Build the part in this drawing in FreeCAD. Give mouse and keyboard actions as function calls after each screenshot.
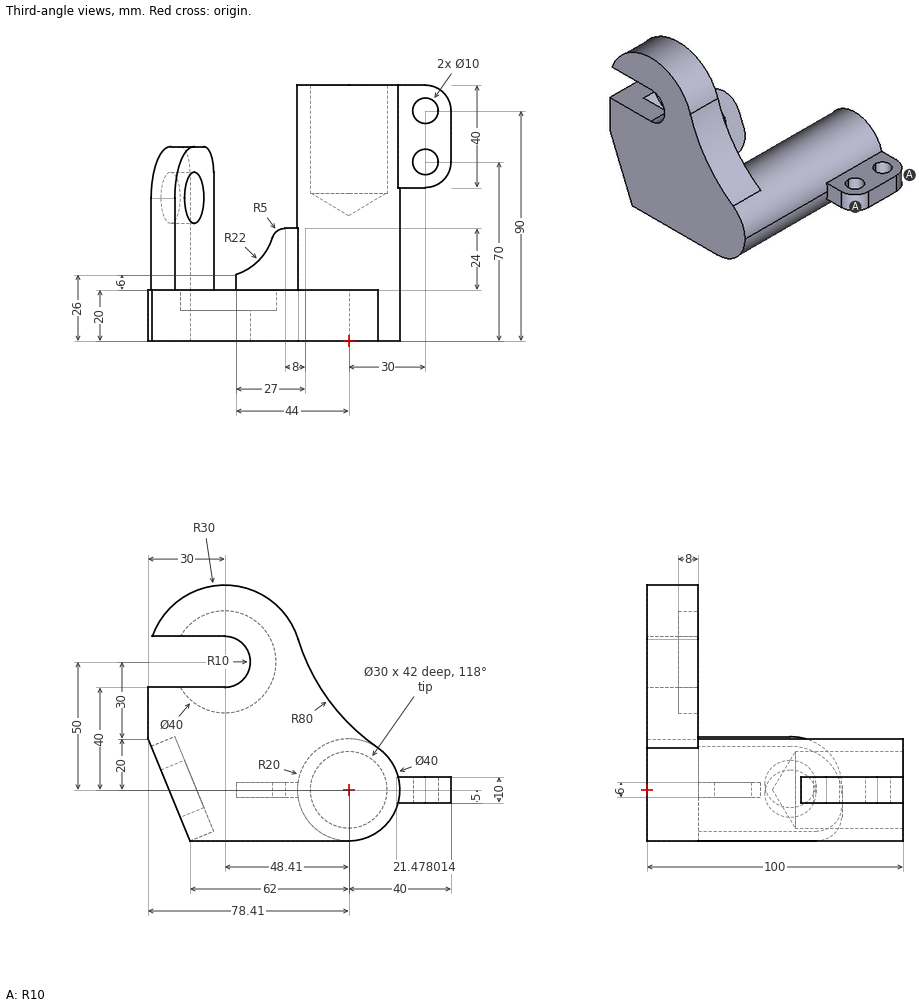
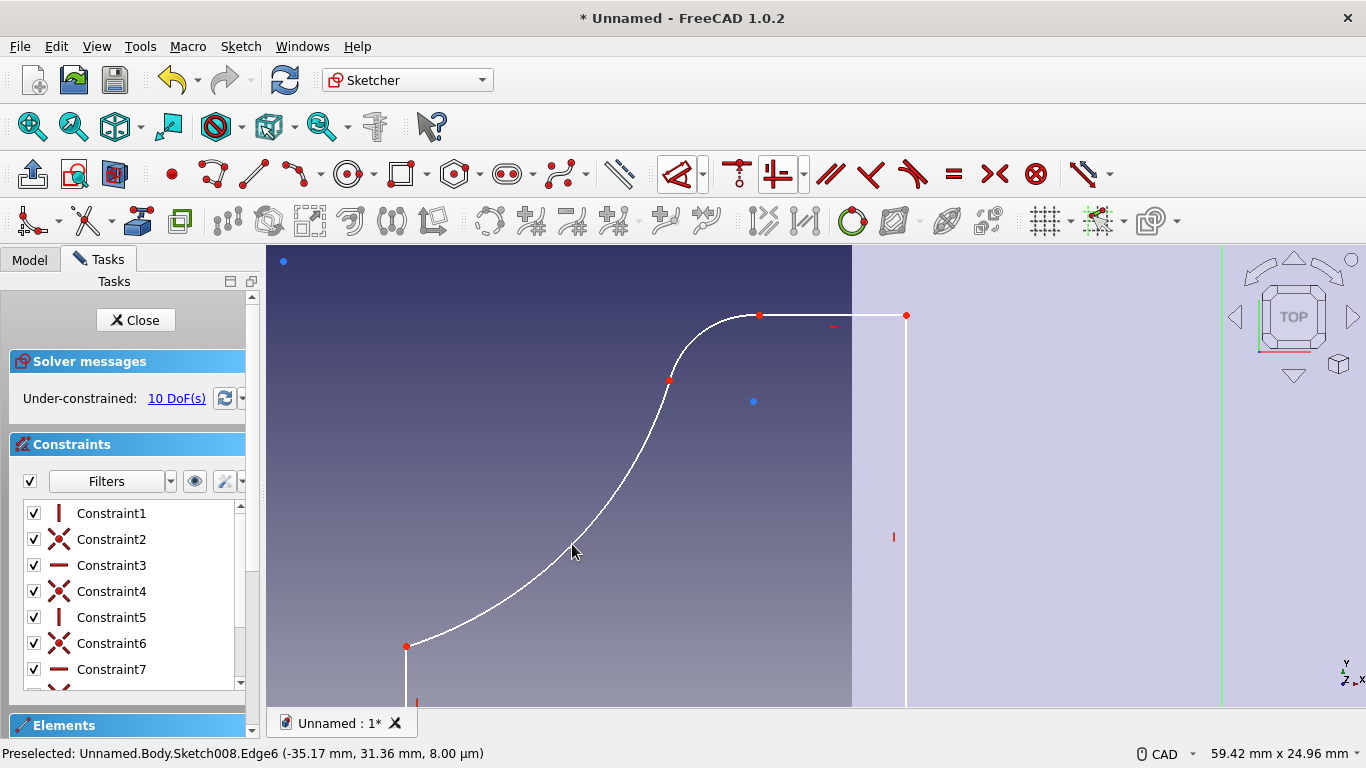
click(862, 315)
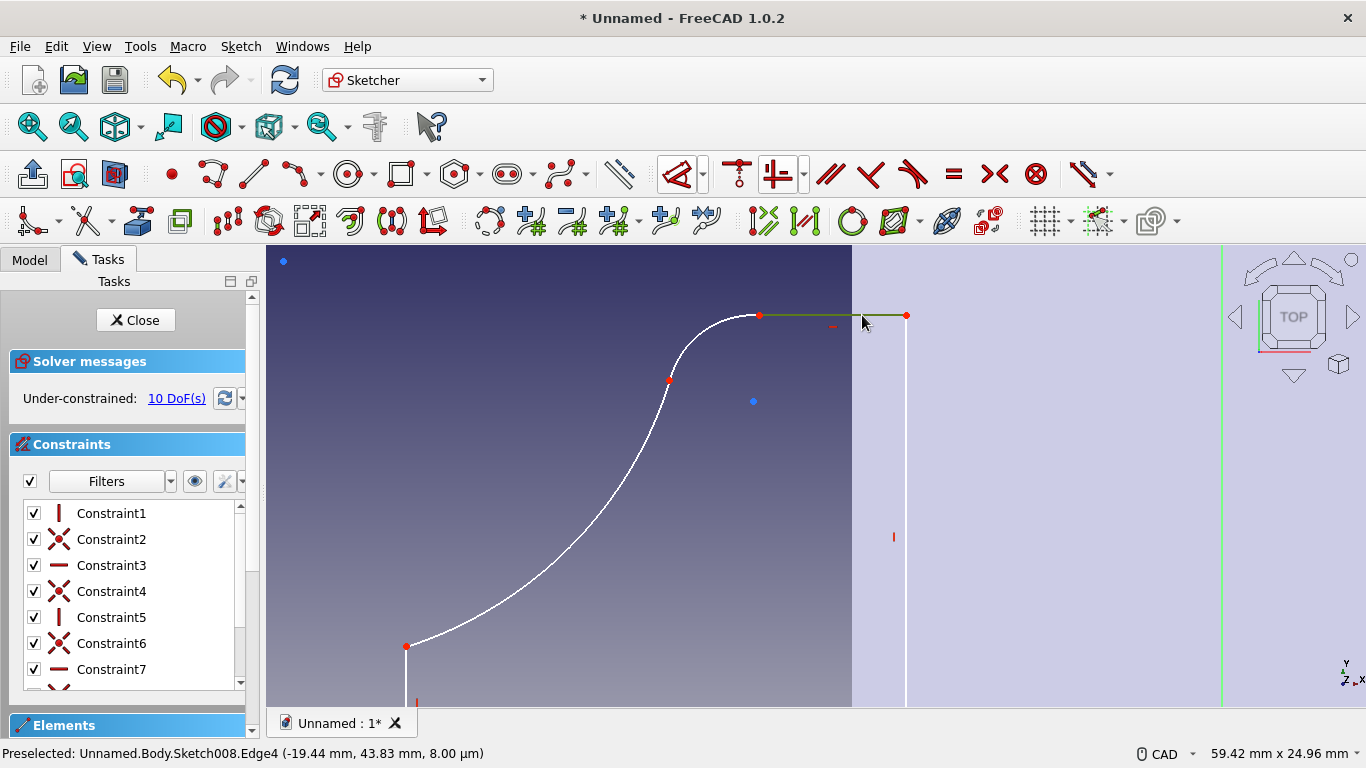
click(724, 320)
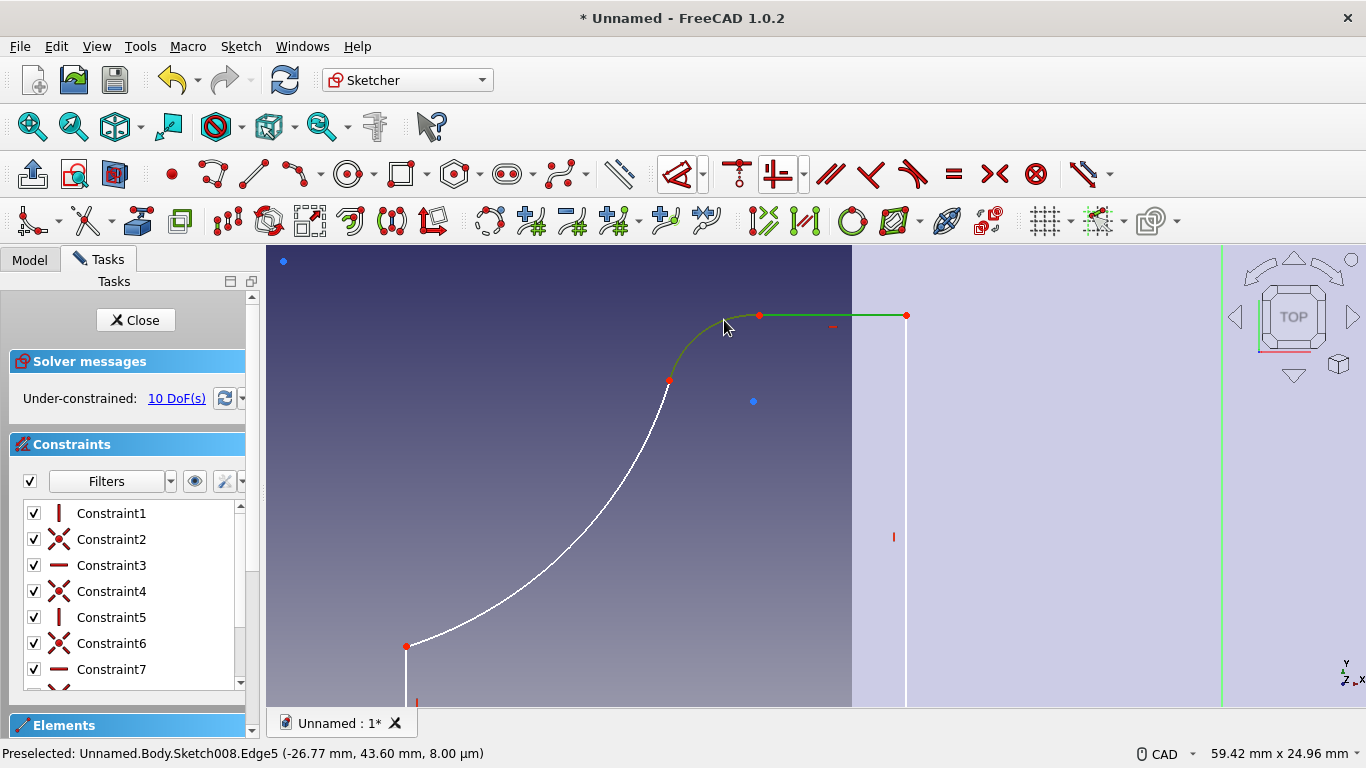
key(t)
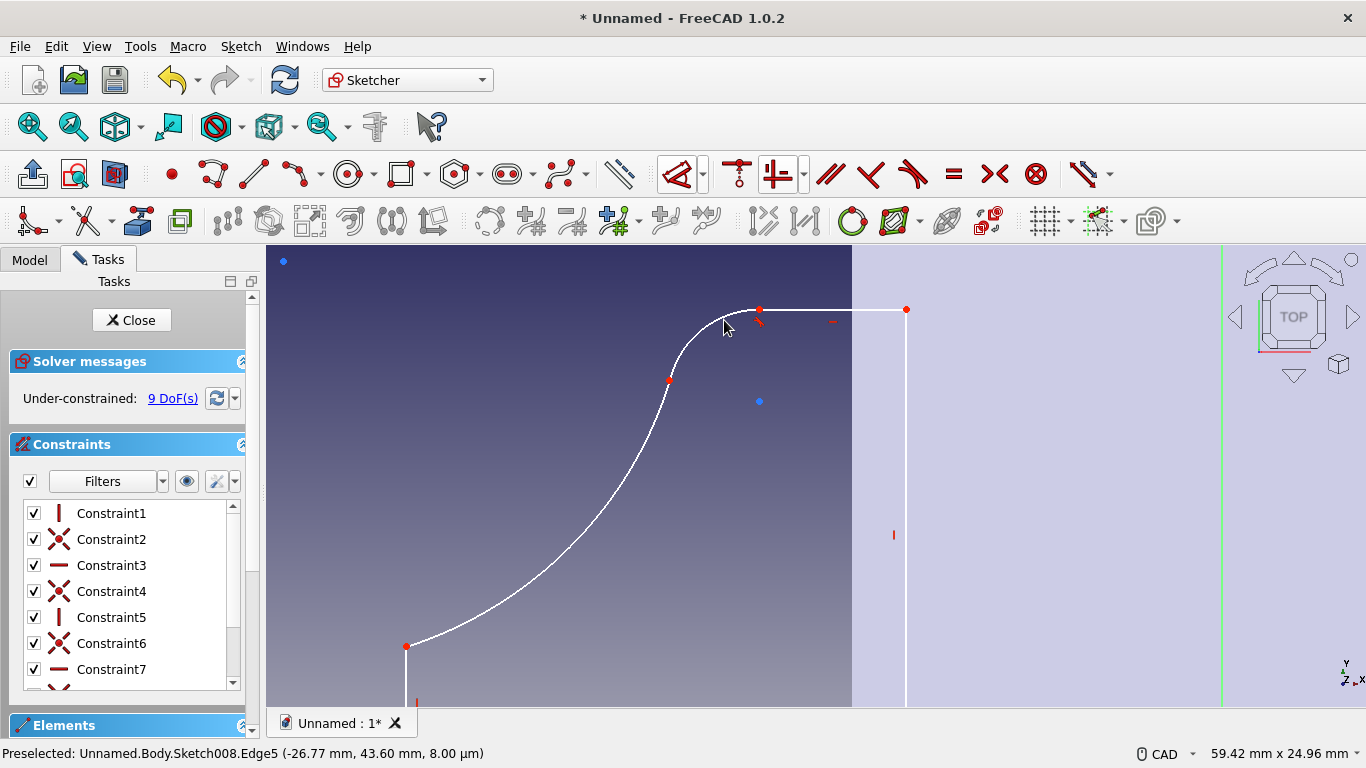
click(724, 317)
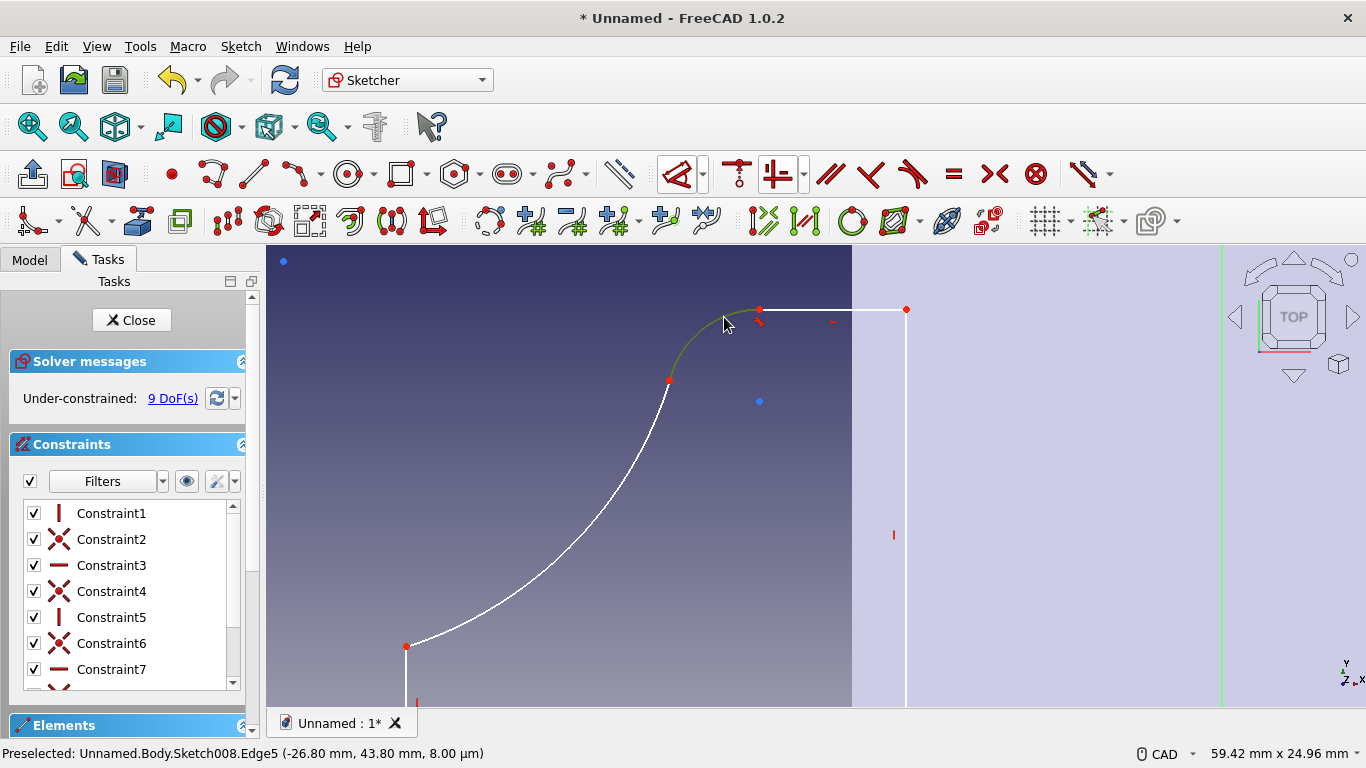
click(511, 596)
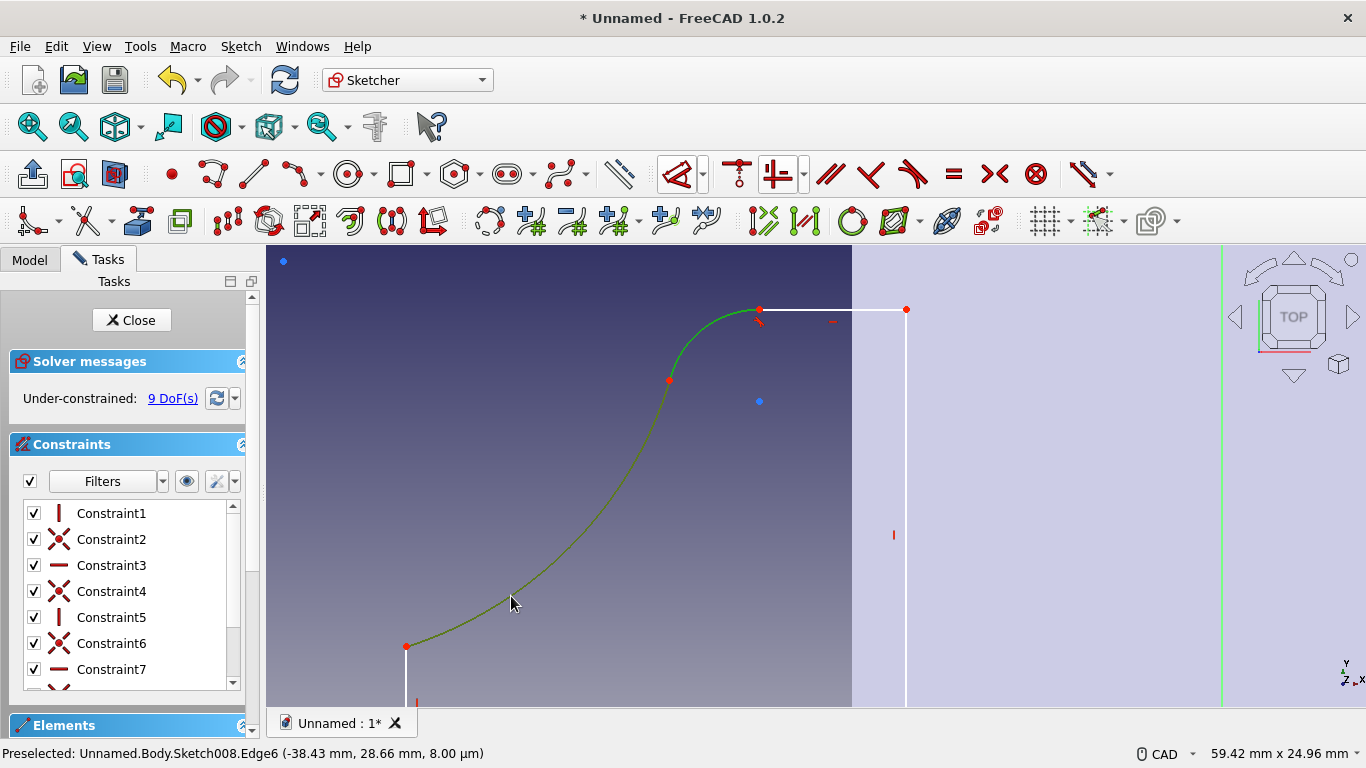
click(913, 174)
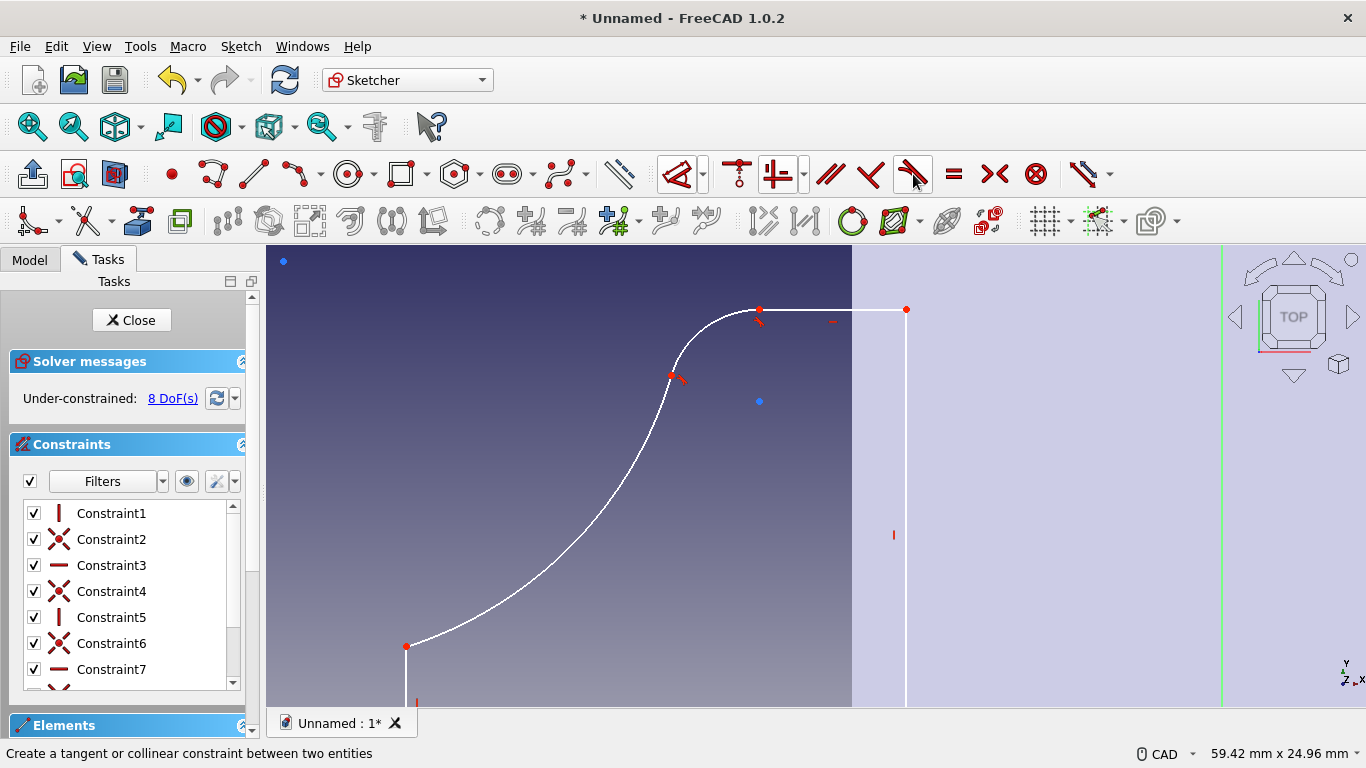
key(d)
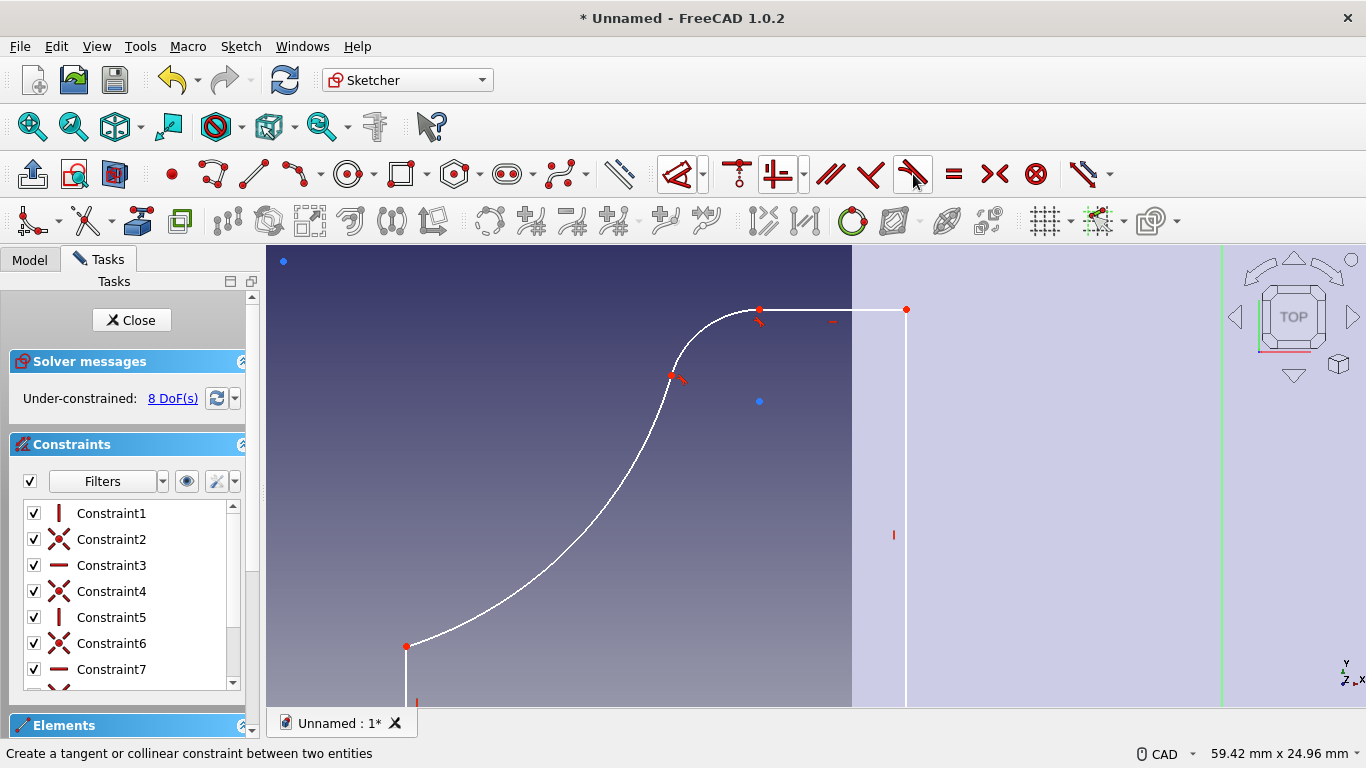
click(725, 317)
click(713, 287)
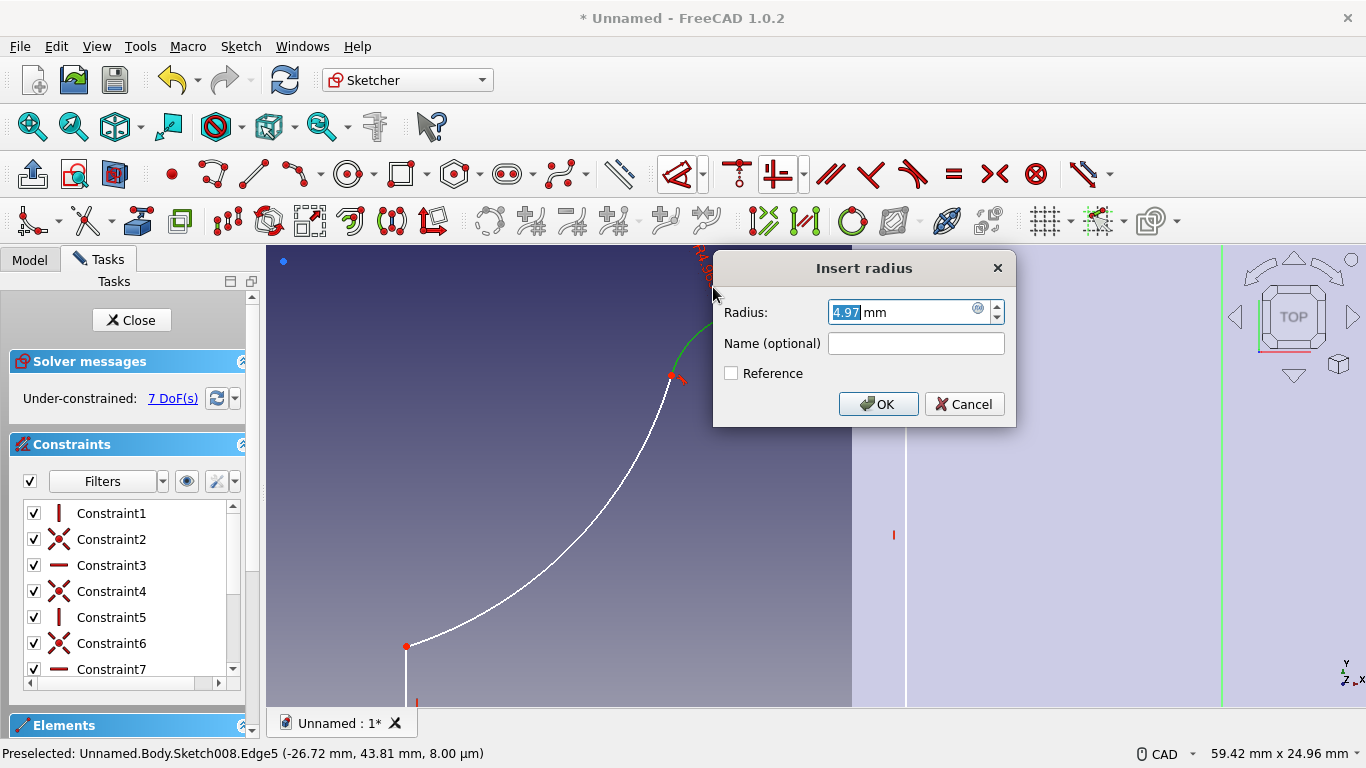
text(5)
key(Return)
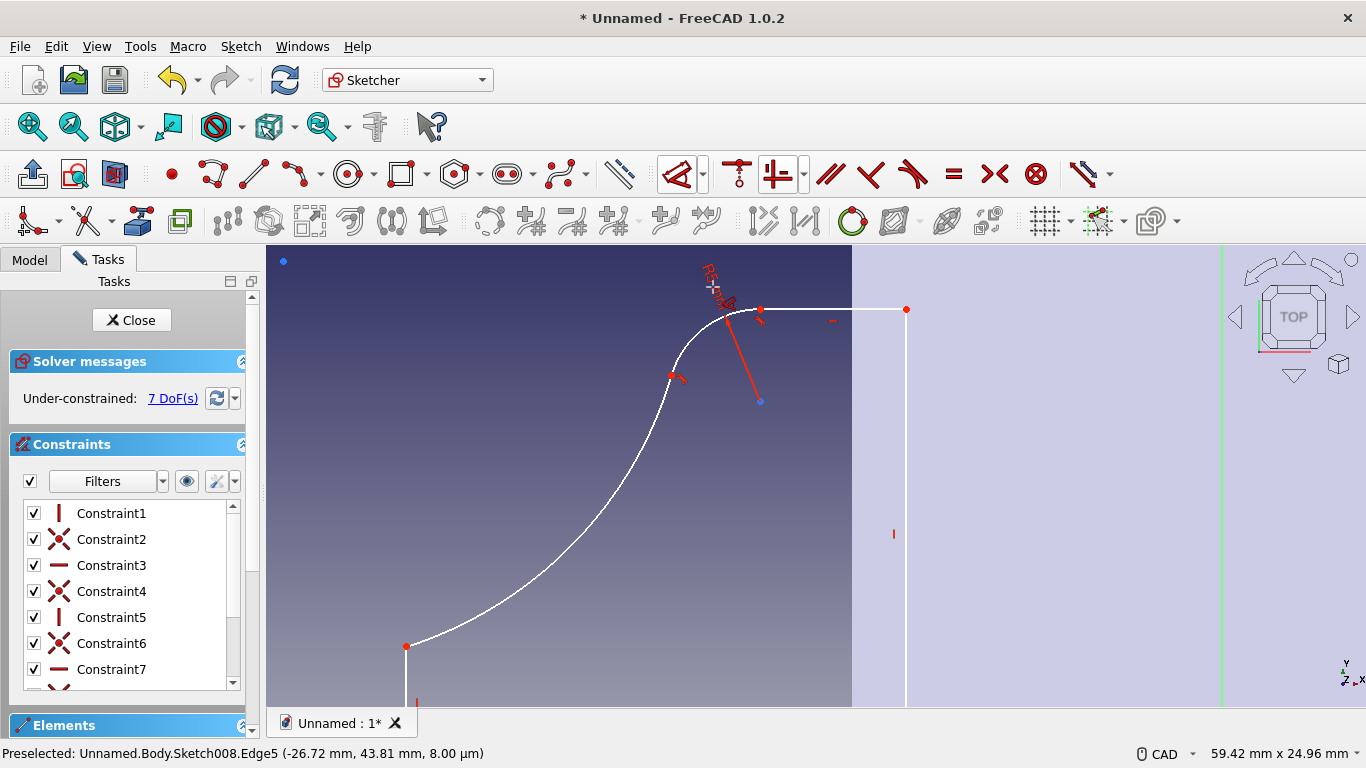
click(512, 595)
click(530, 621)